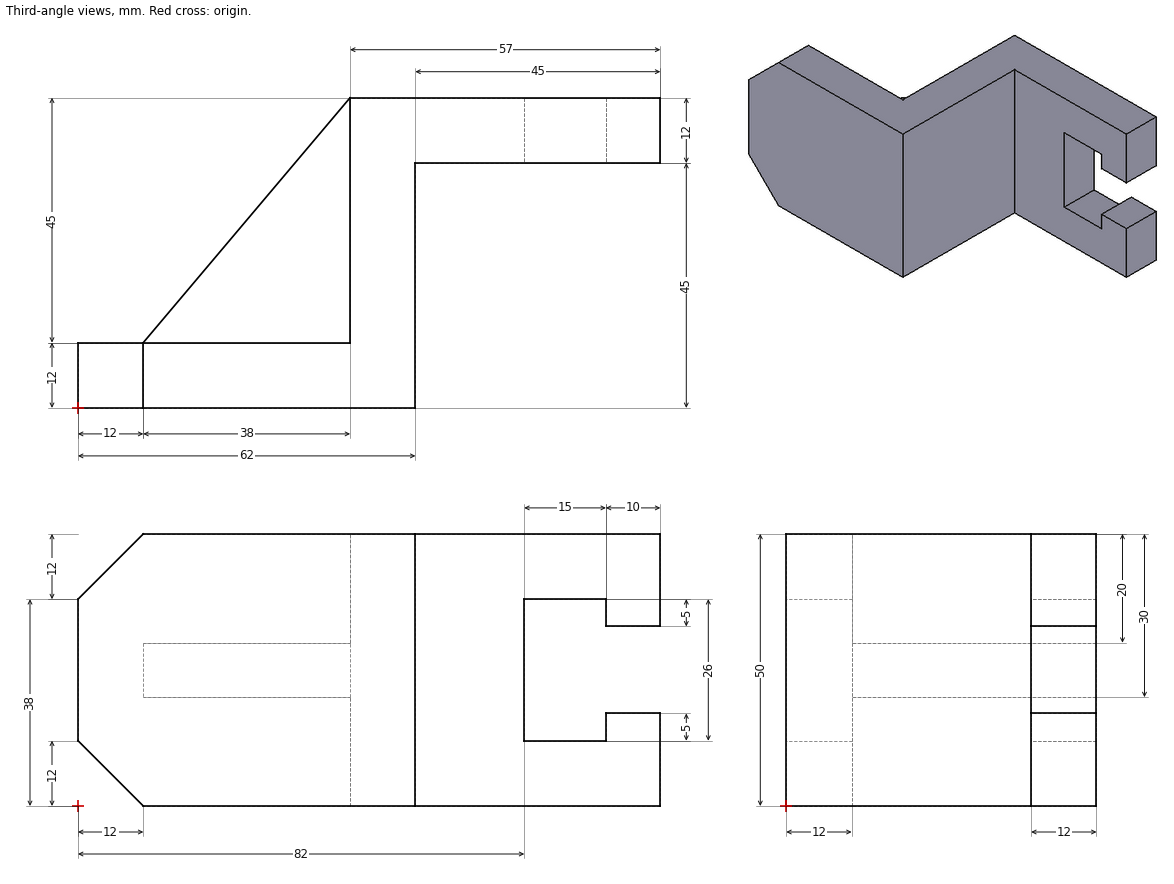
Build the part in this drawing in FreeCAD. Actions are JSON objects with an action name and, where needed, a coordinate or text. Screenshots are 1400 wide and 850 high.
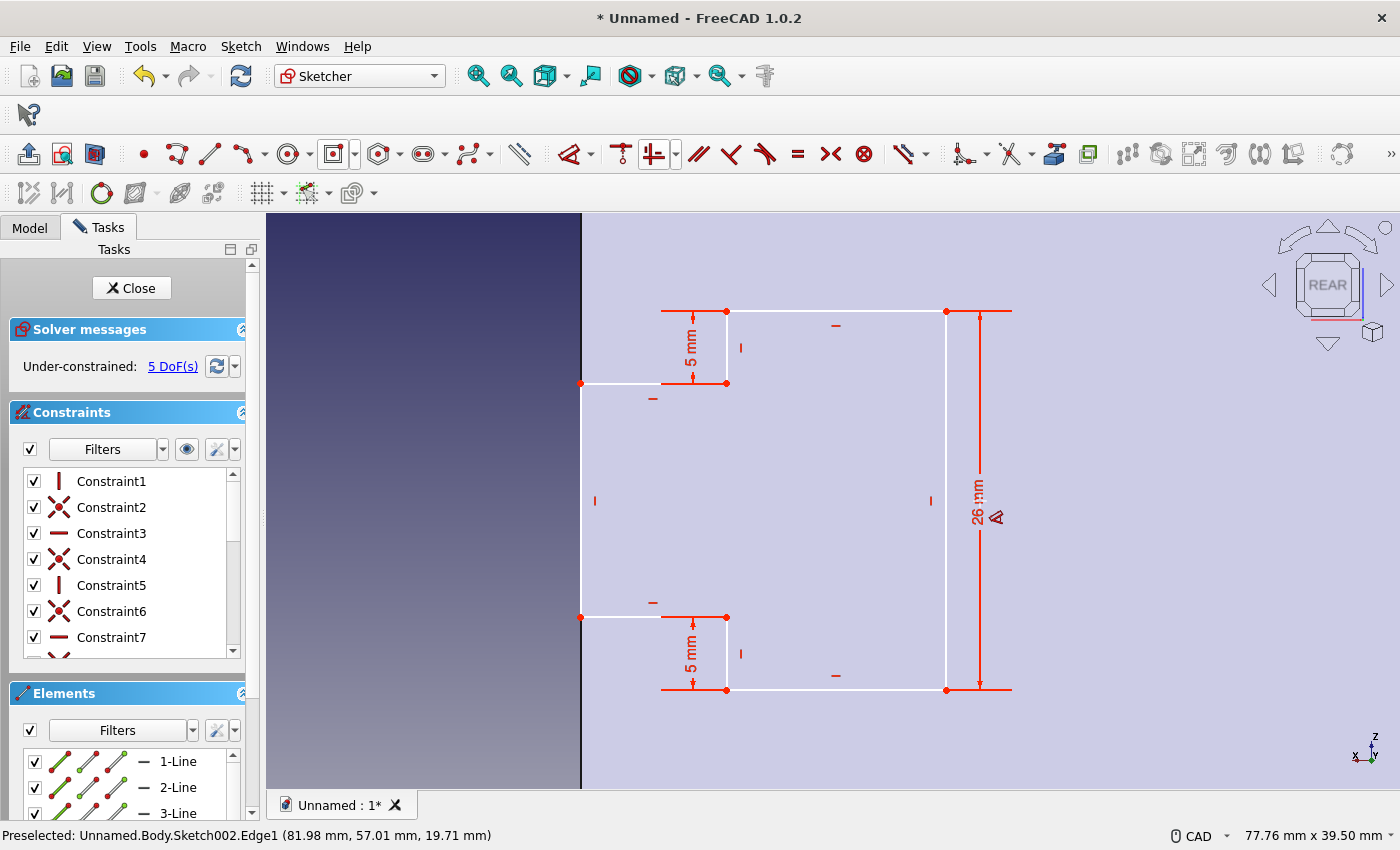
{"action": "left_click", "coordinate": [880, 311]}
{"action": "left_click", "coordinate": [837, 277]}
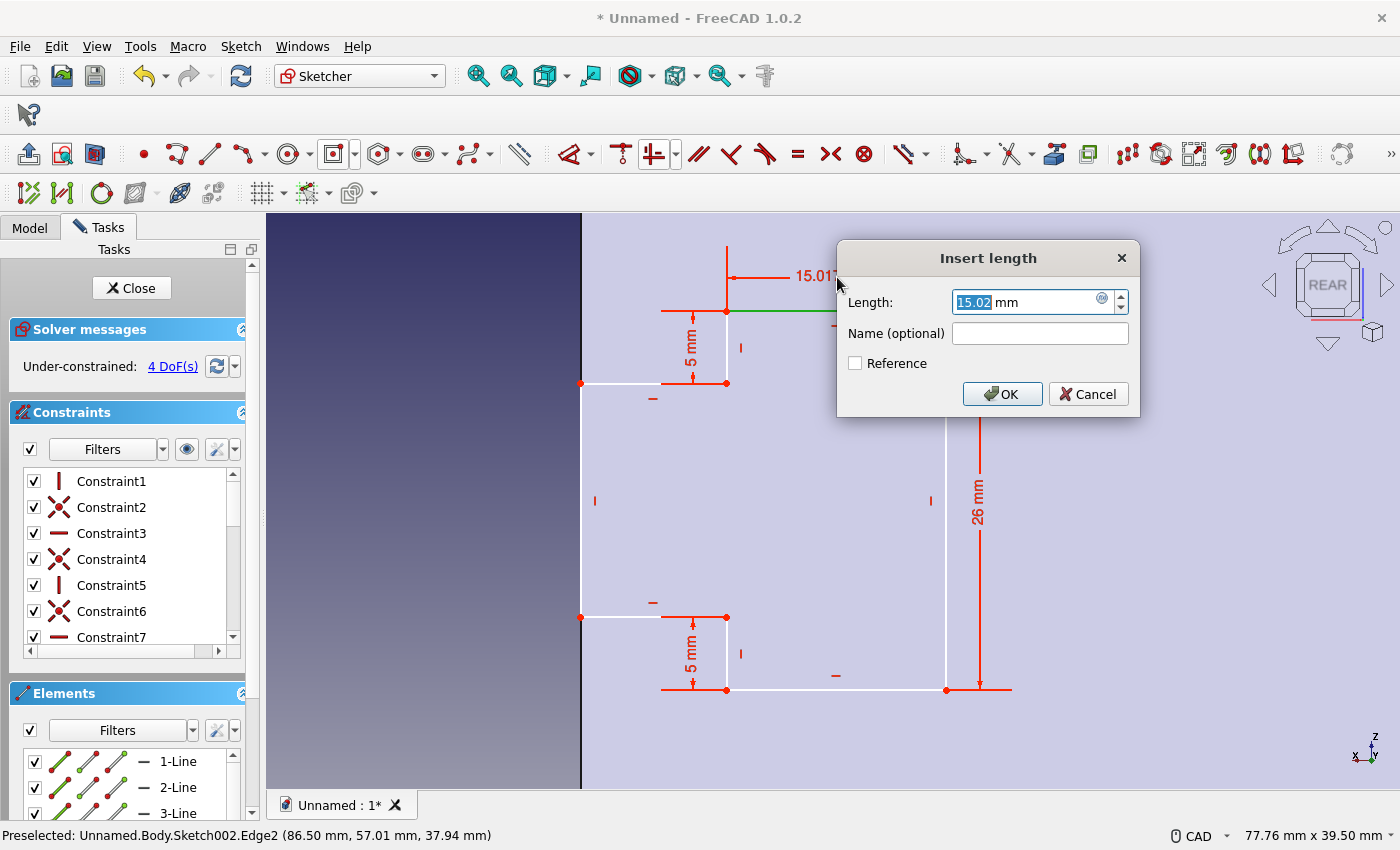
{"action": "type", "text": "15"}
{"action": "key", "text": "Return"}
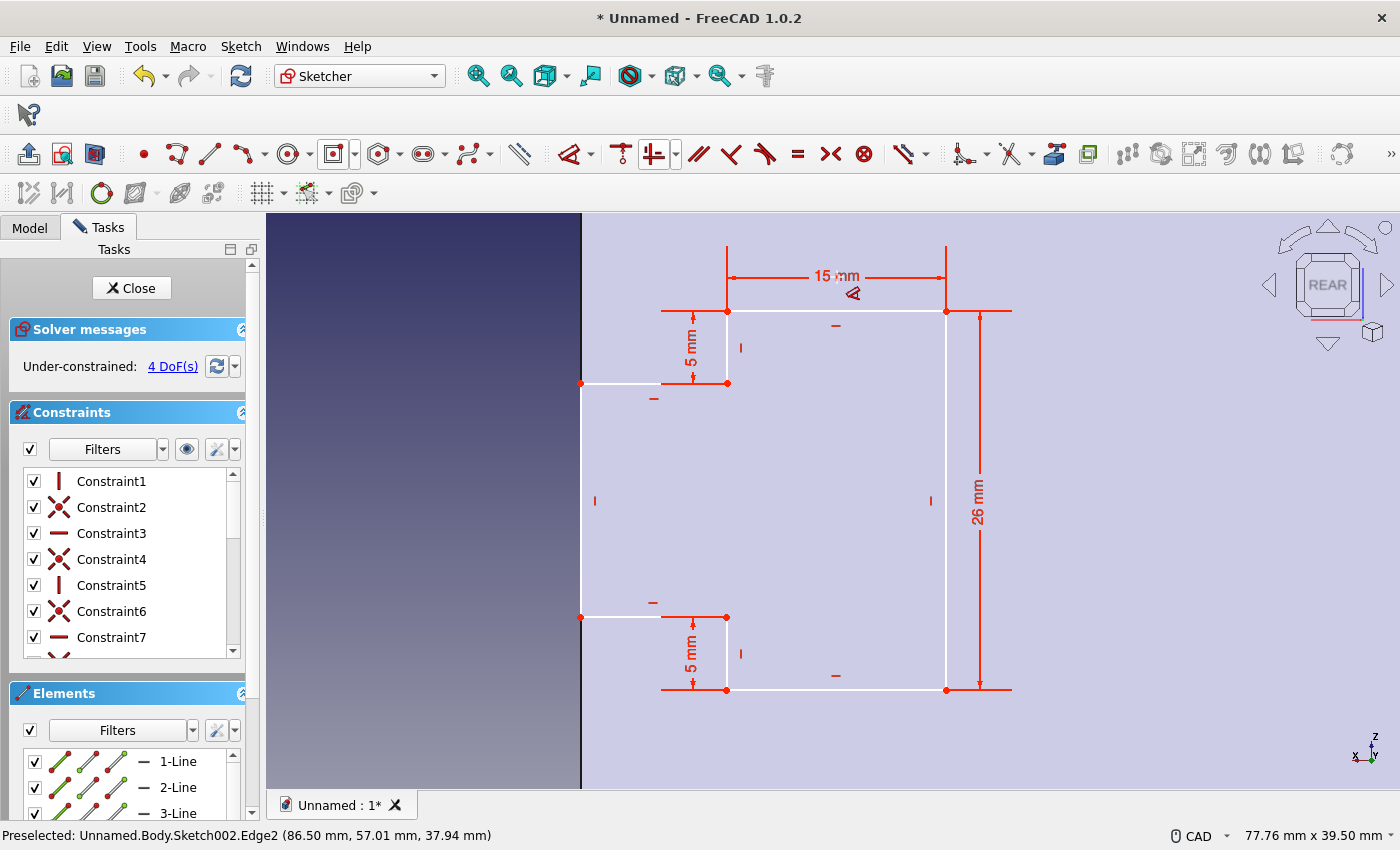
{"action": "left_click", "coordinate": [683, 384]}
{"action": "left_click", "coordinate": [620, 350]}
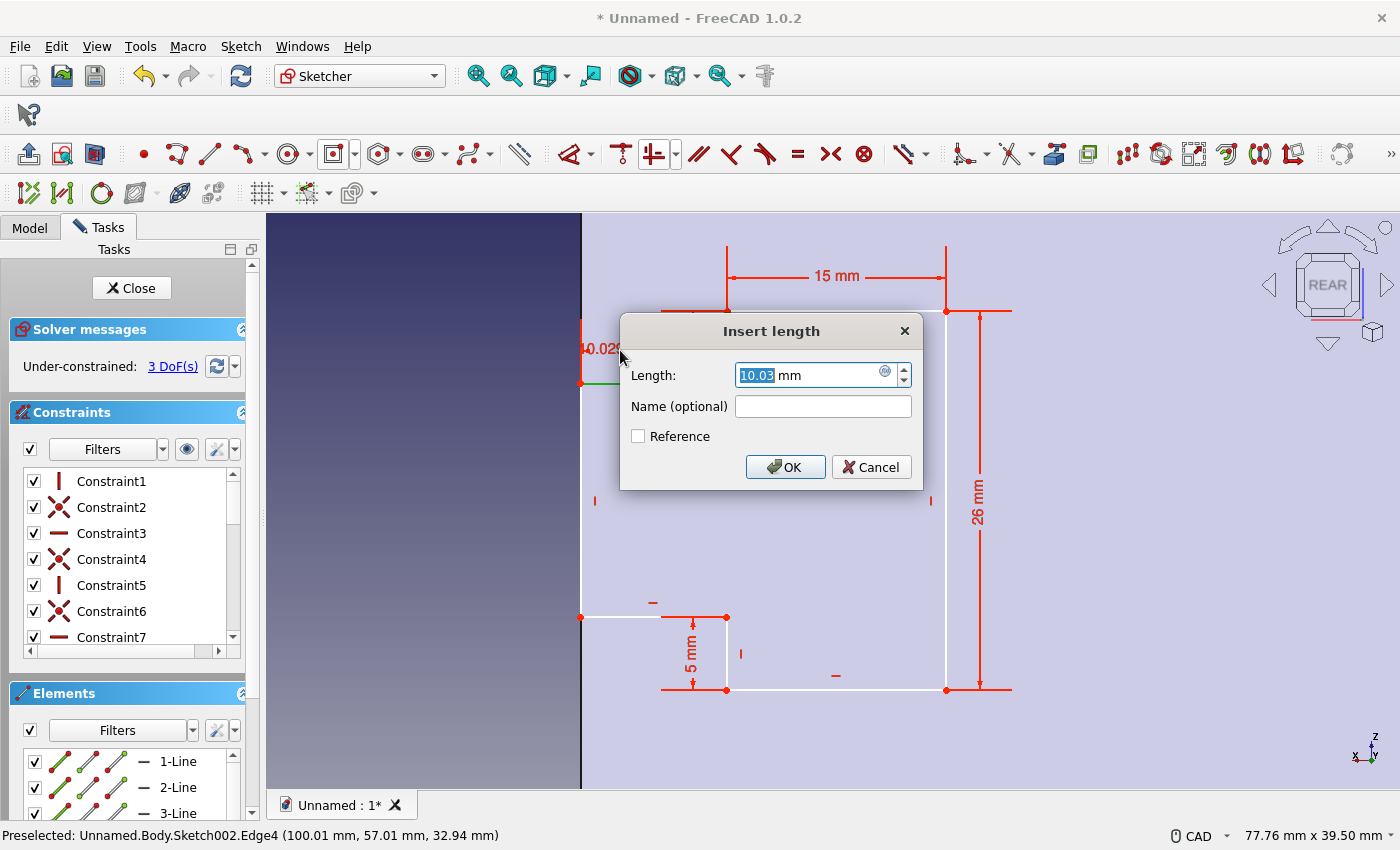
{"action": "type", "text": "10"}
{"action": "key", "text": "Return"}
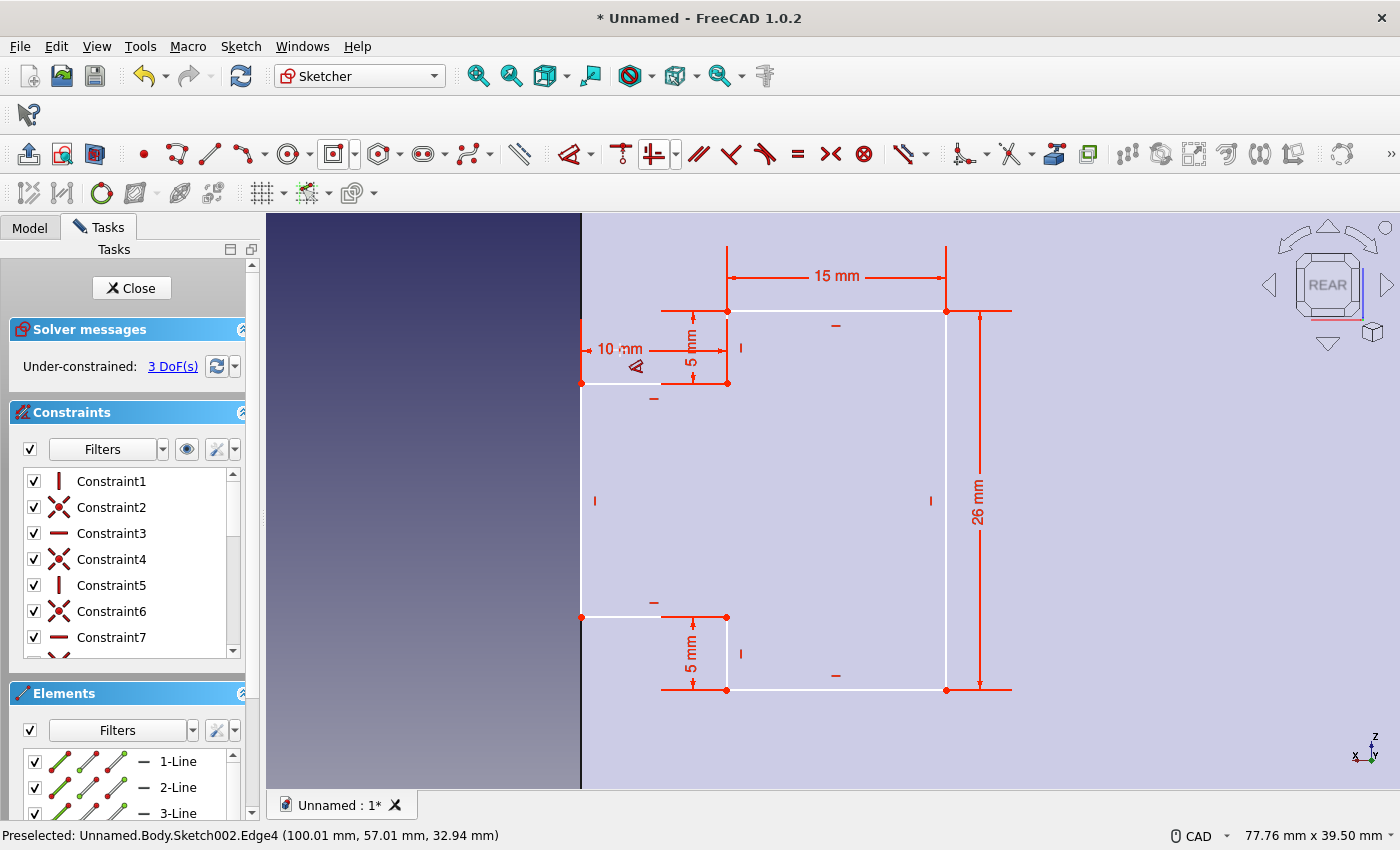
{"action": "left_click", "coordinate": [625, 617]}
{"action": "left_click", "coordinate": [621, 651]}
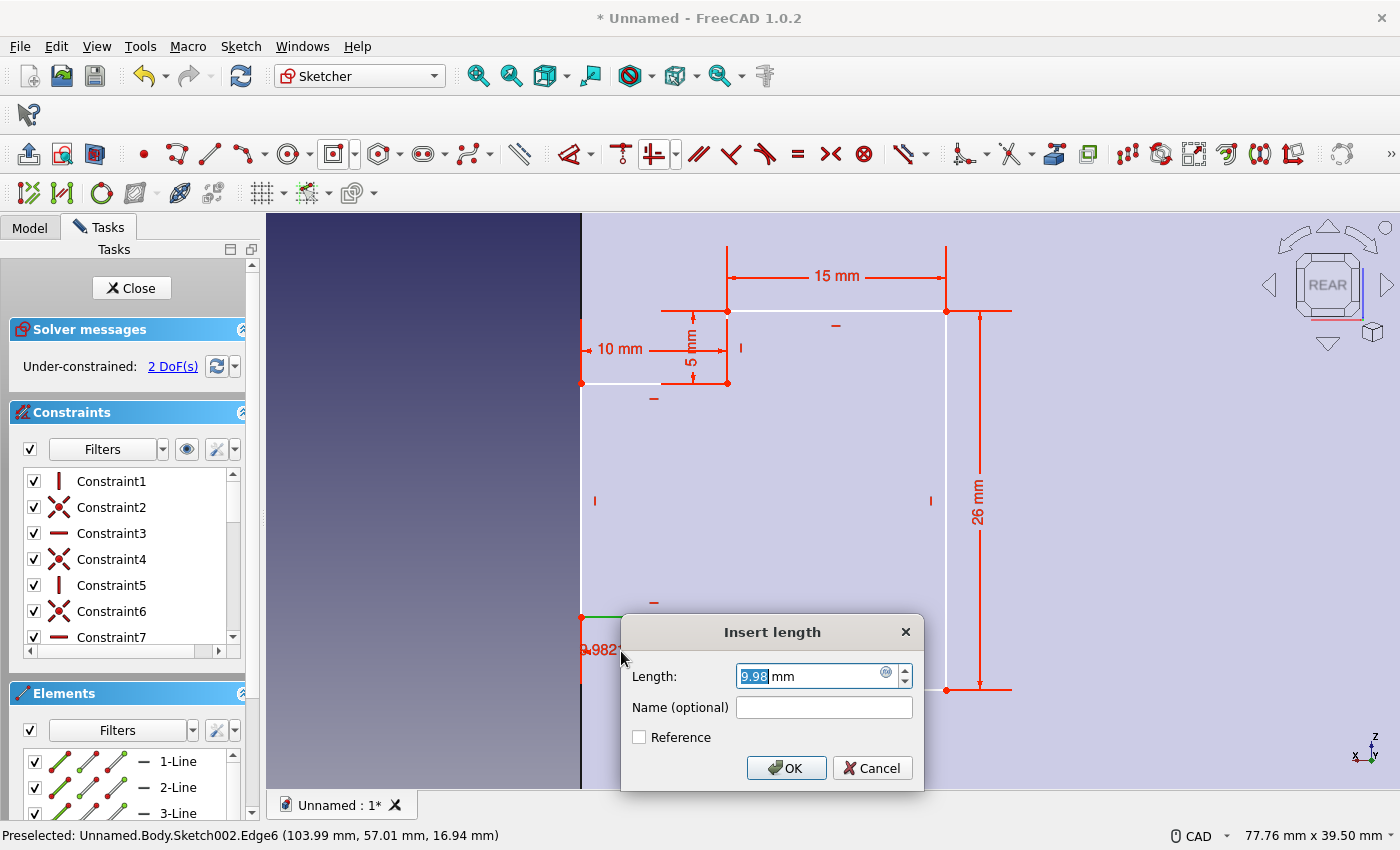
{"action": "type", "text": "10"}
{"action": "key", "text": "Return"}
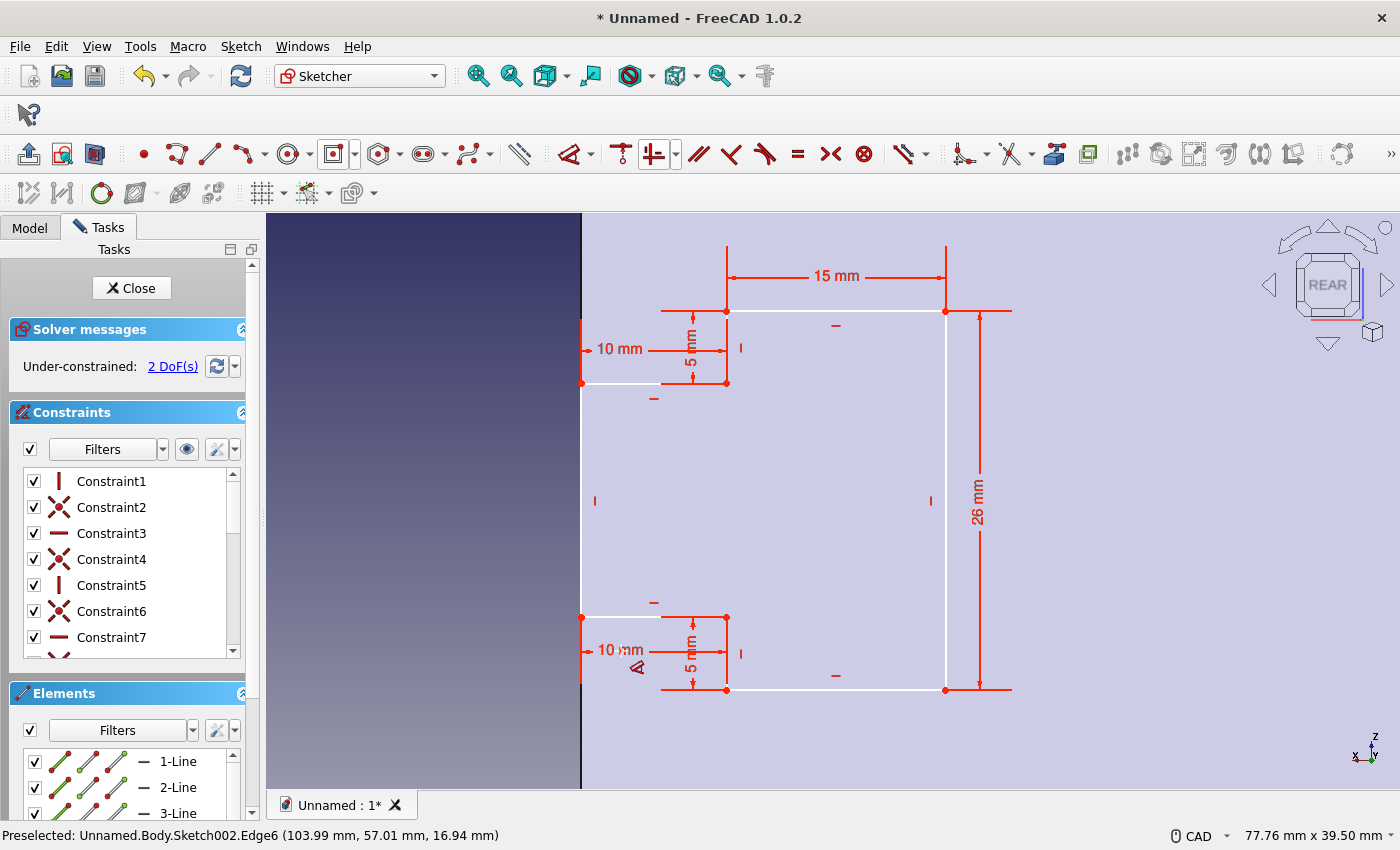
{"action": "left_click", "coordinate": [946, 690]}
{"action": "left_click", "coordinate": [1090, 656]}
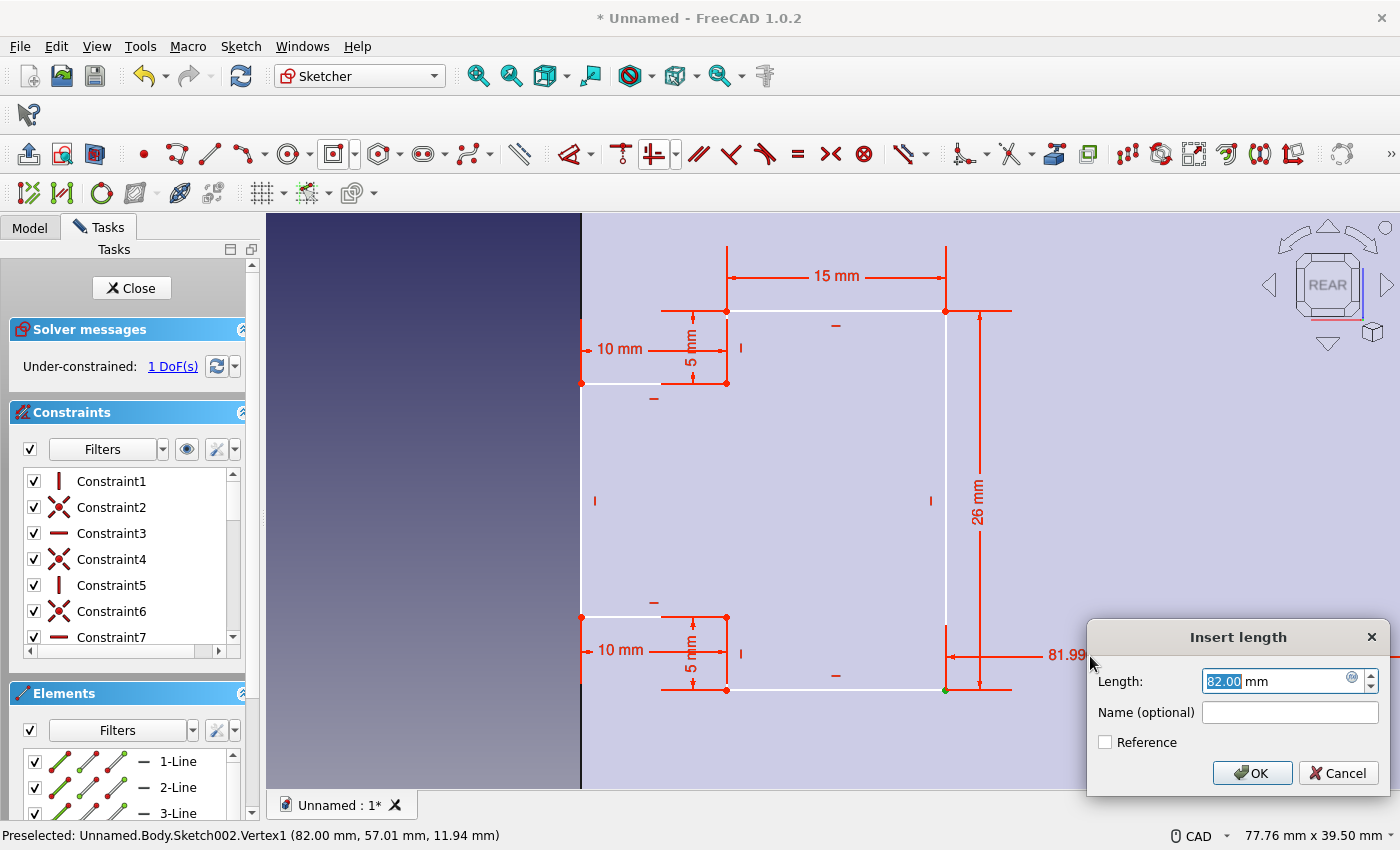
{"action": "type", "text": "82"}
{"action": "key", "text": "Return"}